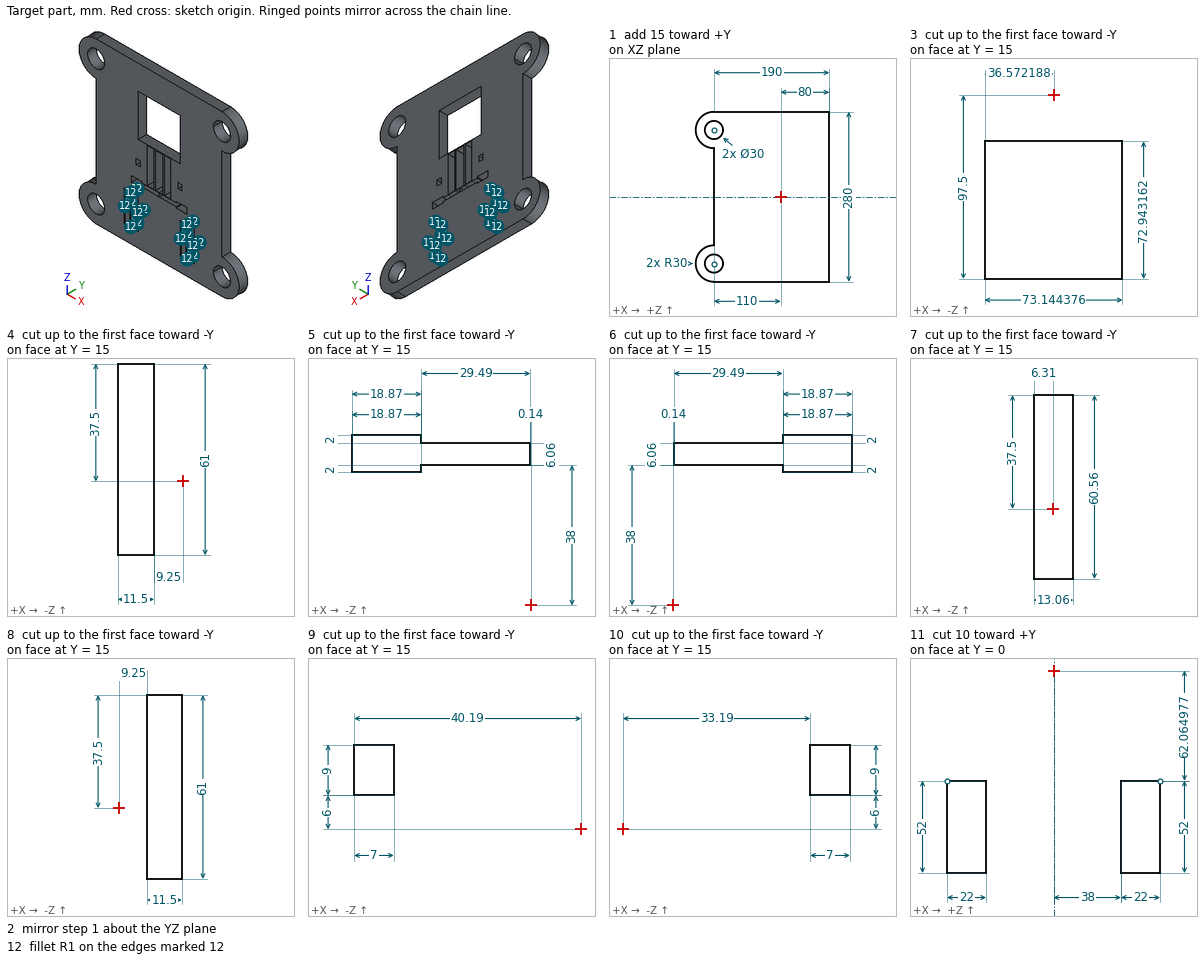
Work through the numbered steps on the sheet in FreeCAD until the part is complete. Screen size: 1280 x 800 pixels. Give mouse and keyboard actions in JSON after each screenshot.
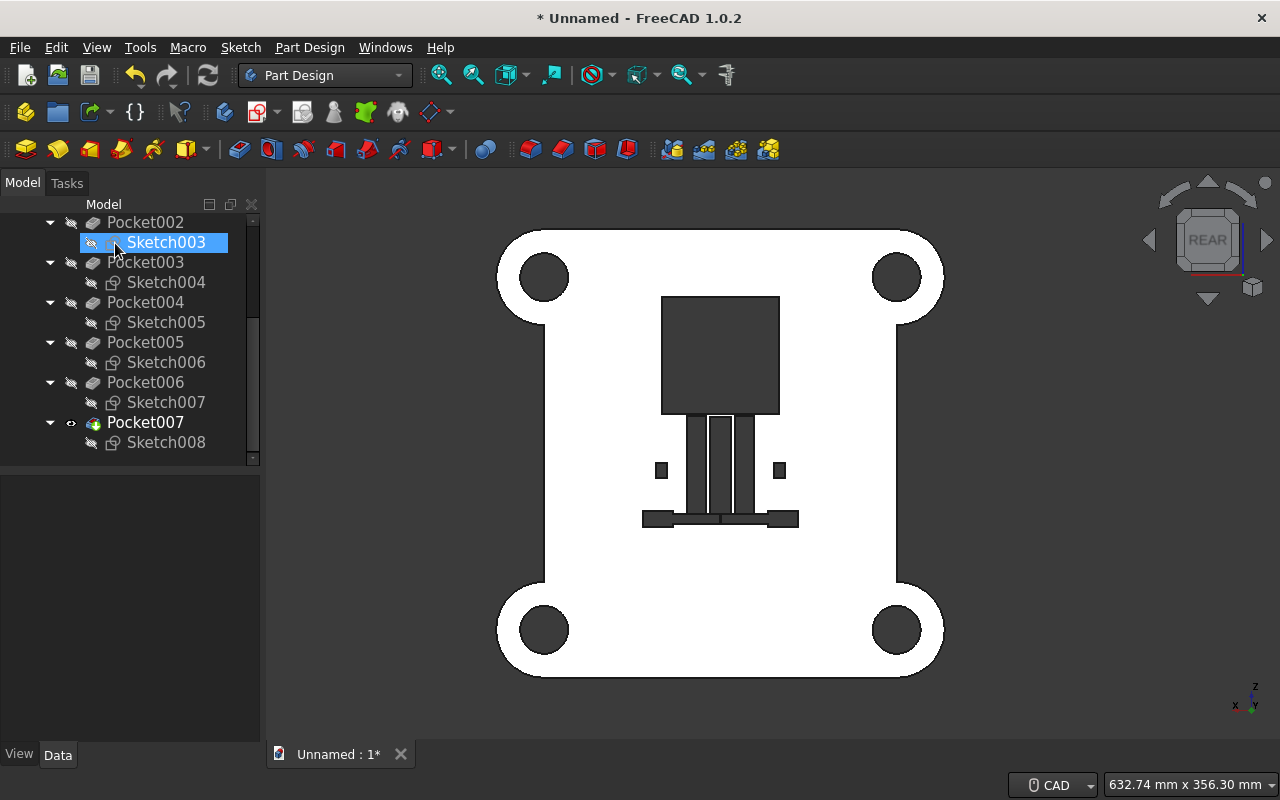
{"action": "key", "text": "0"}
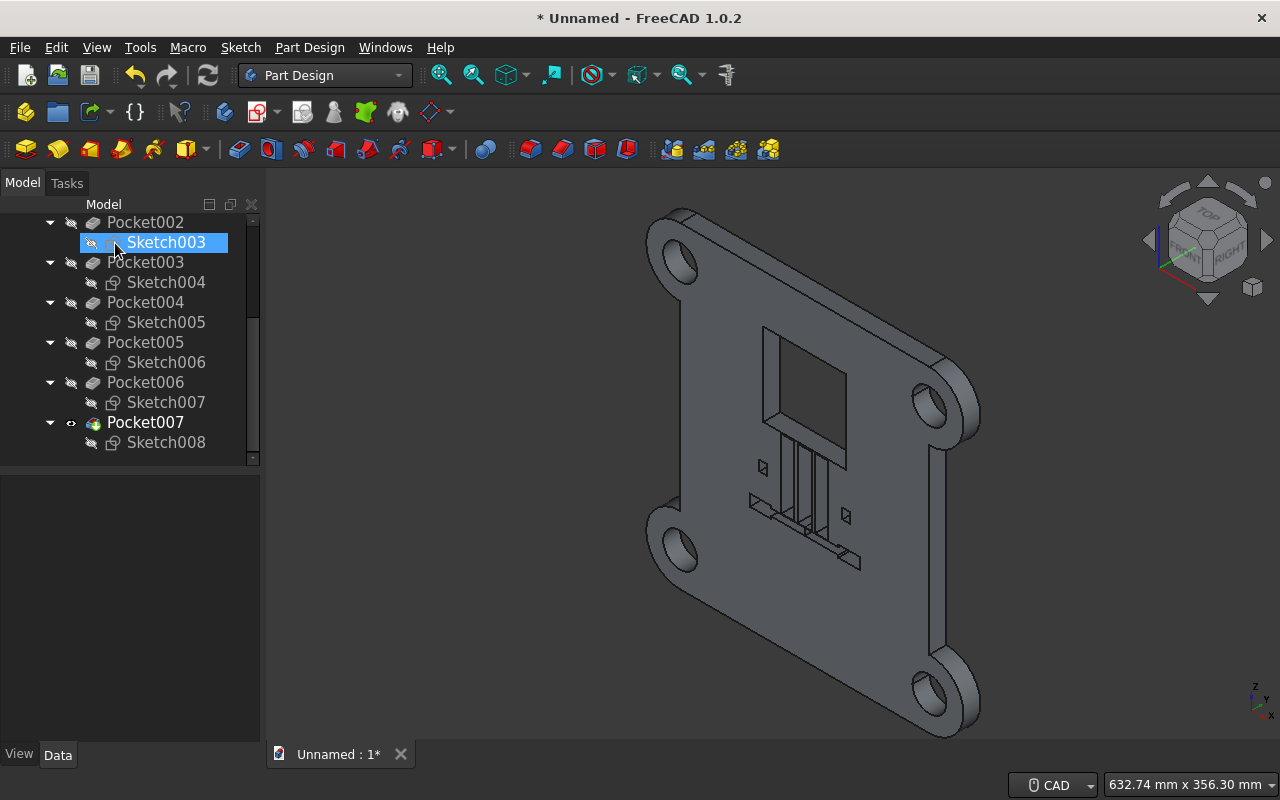
{"action": "left_click", "coordinate": [442, 76]}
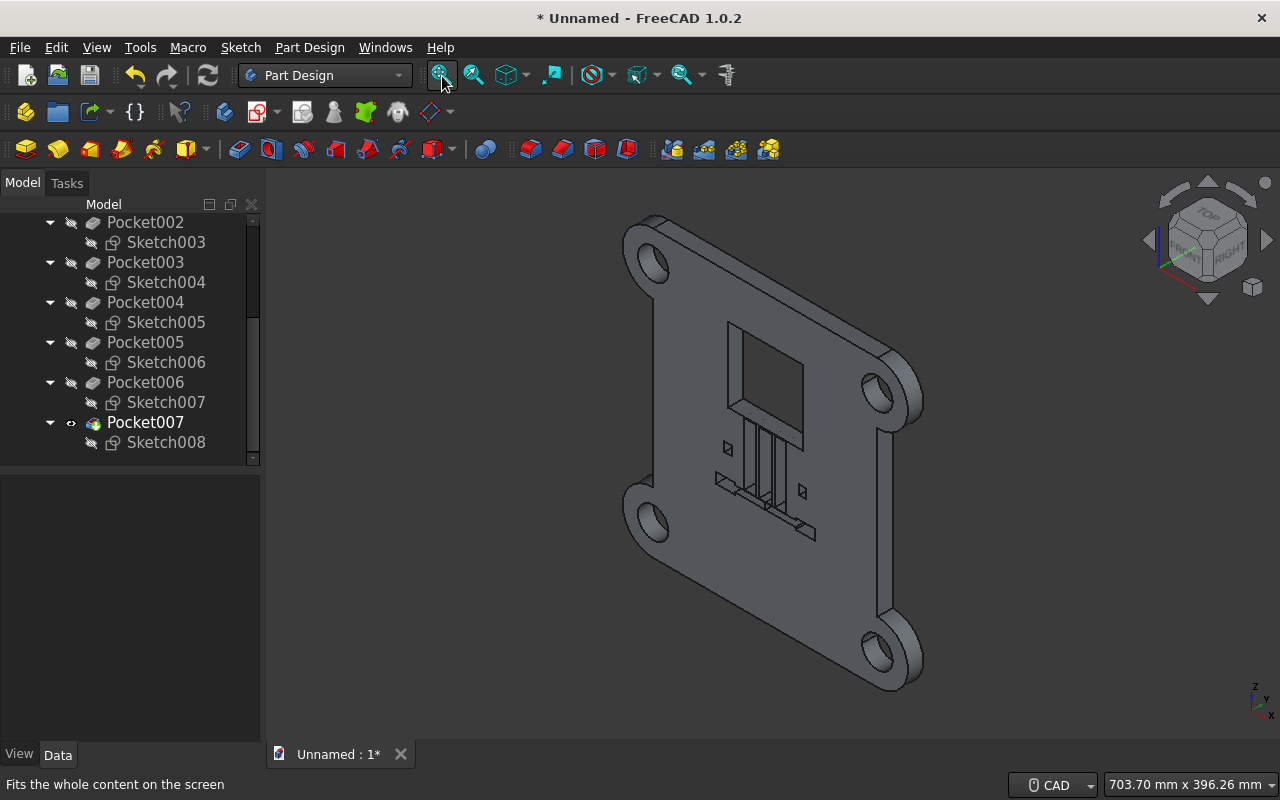
{"action": "left_click", "coordinate": [765, 551]}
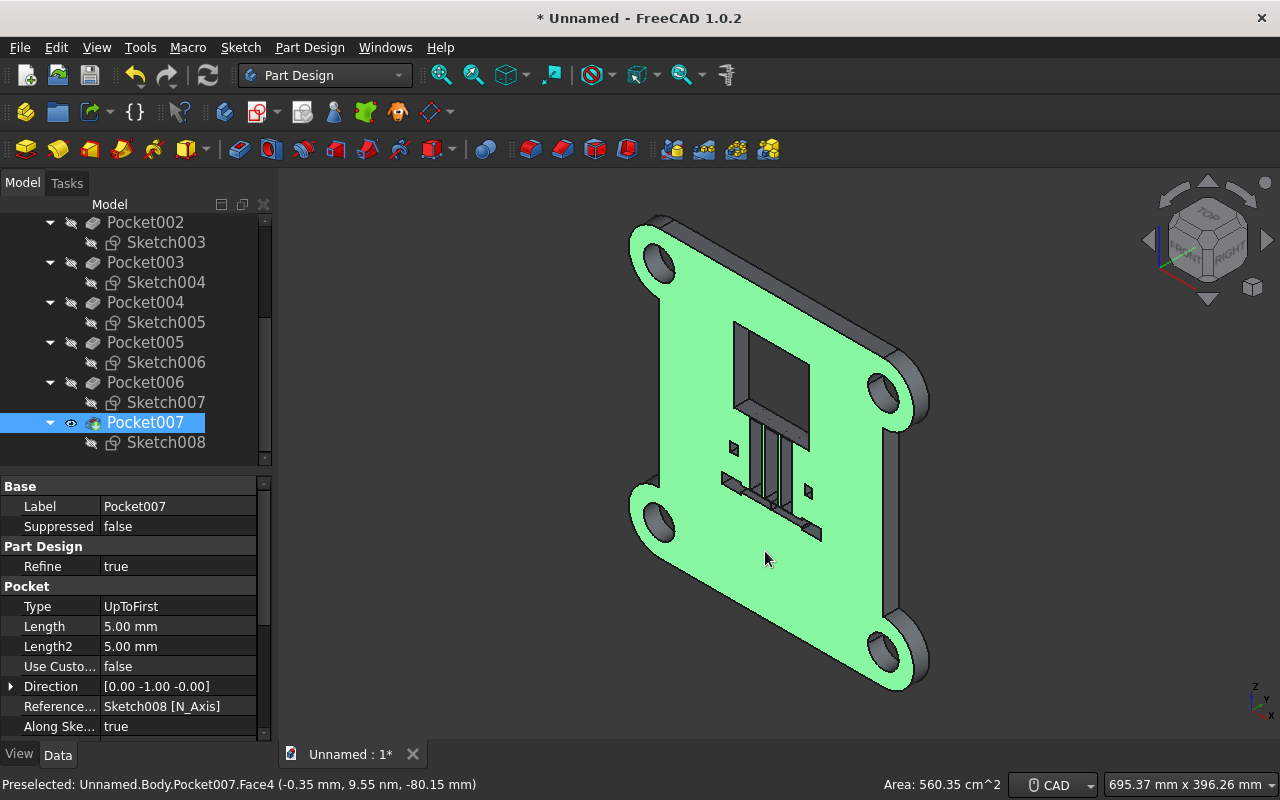
{"action": "left_click", "coordinate": [258, 112]}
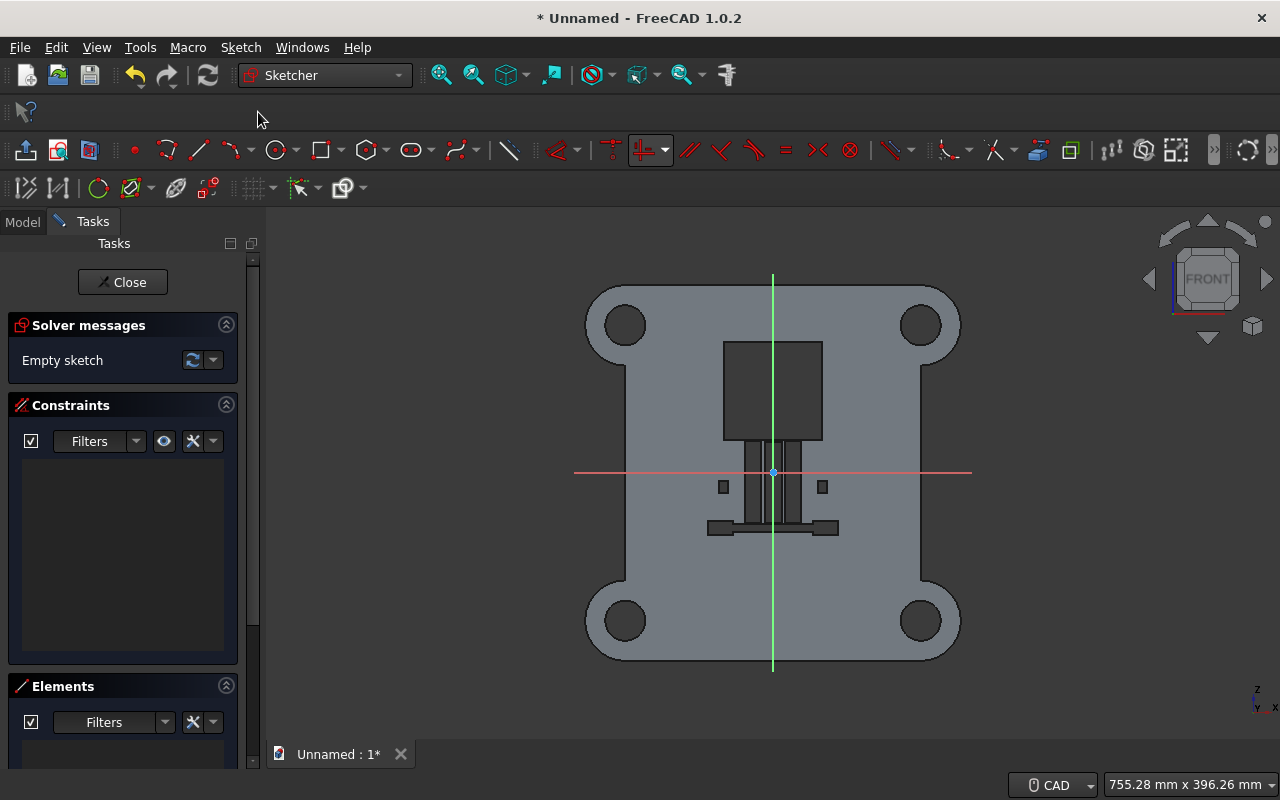
{"action": "scroll", "coordinate": [829, 612], "scroll_direction": "up", "scroll_amount": 4}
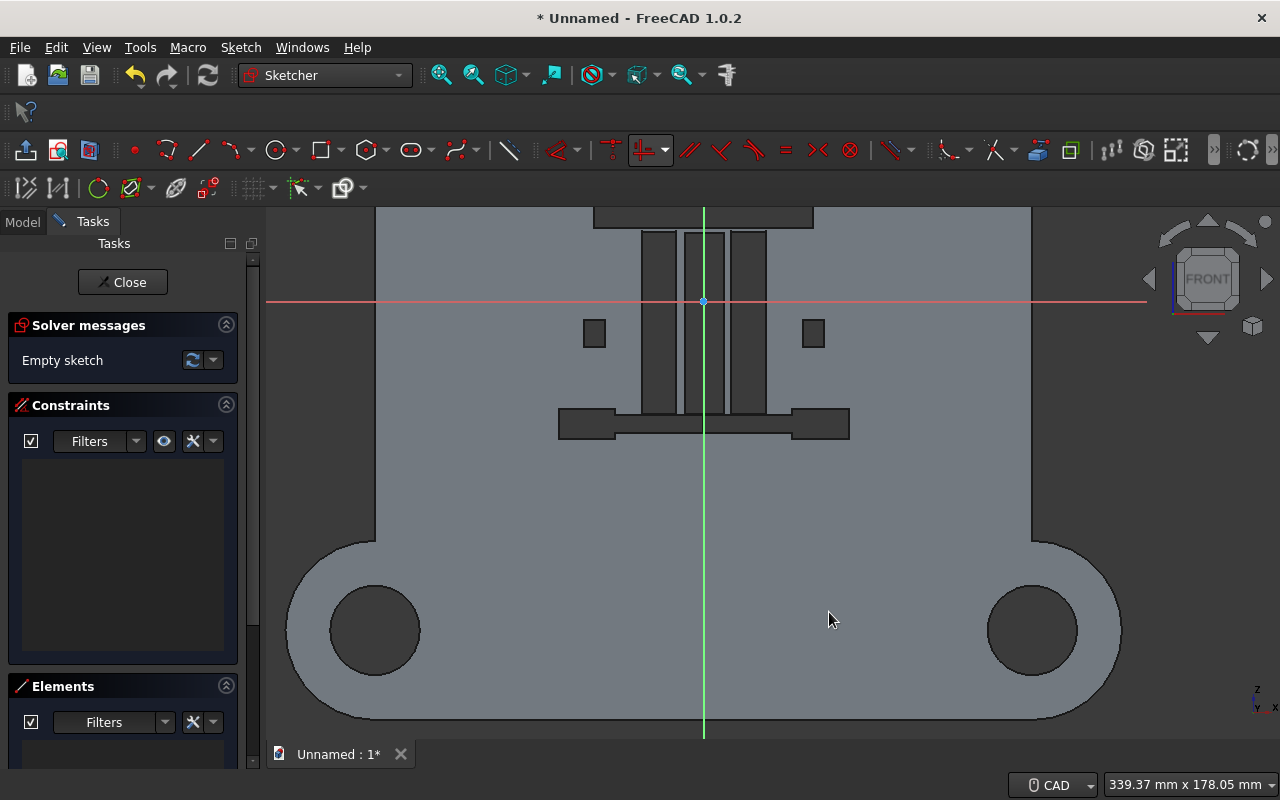
{"action": "left_click", "coordinate": [322, 150]}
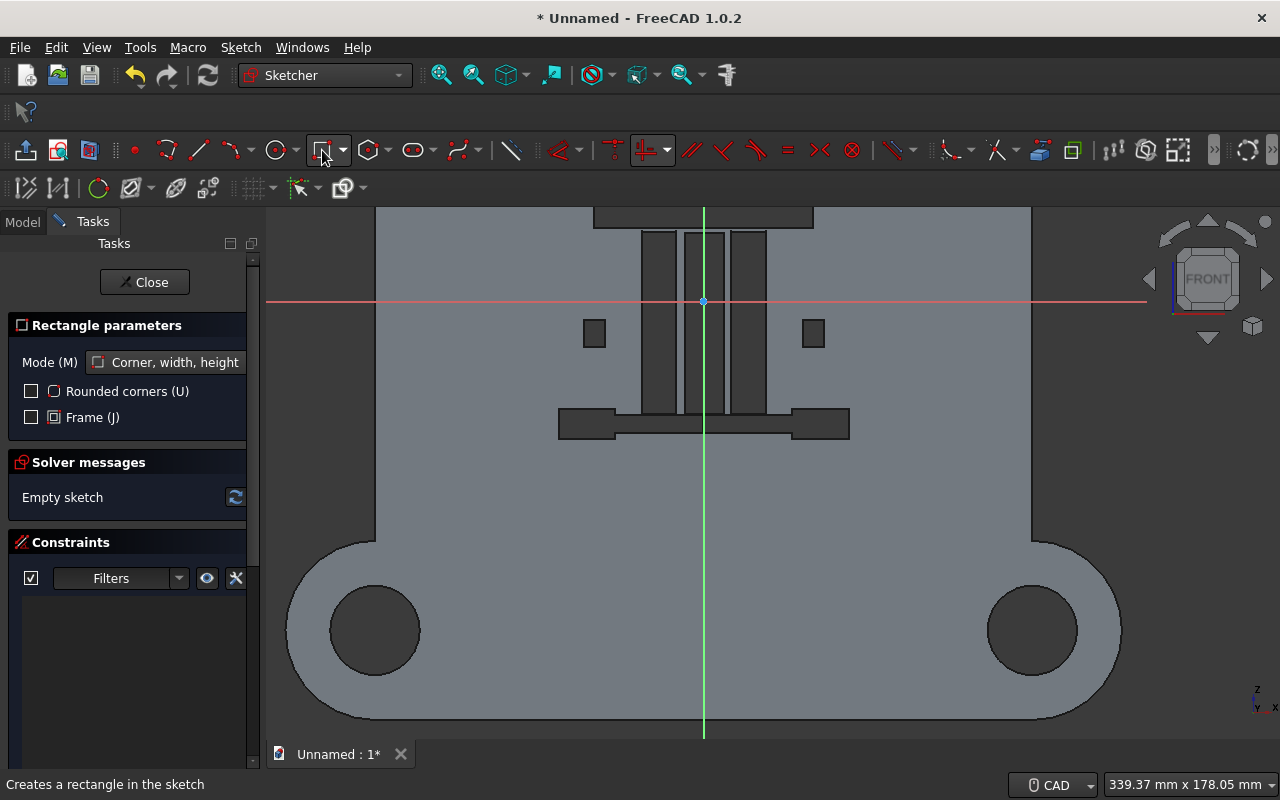
{"action": "left_click", "coordinate": [817, 487]}
{"action": "mouse_move", "coordinate": [883, 643]}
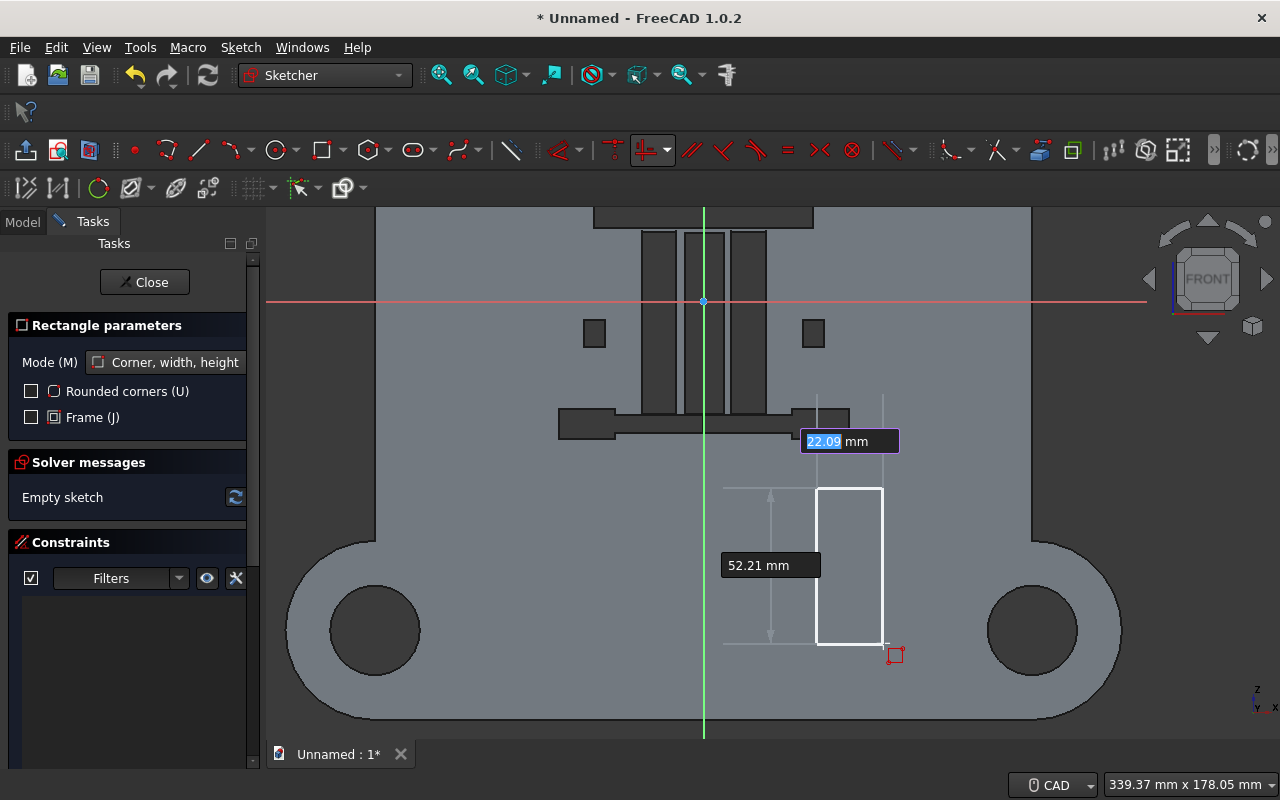
{"action": "type", "text": "22"}
{"action": "key", "text": "Tab"}
{"action": "type", "text": "52"}
{"action": "key", "text": "Return"}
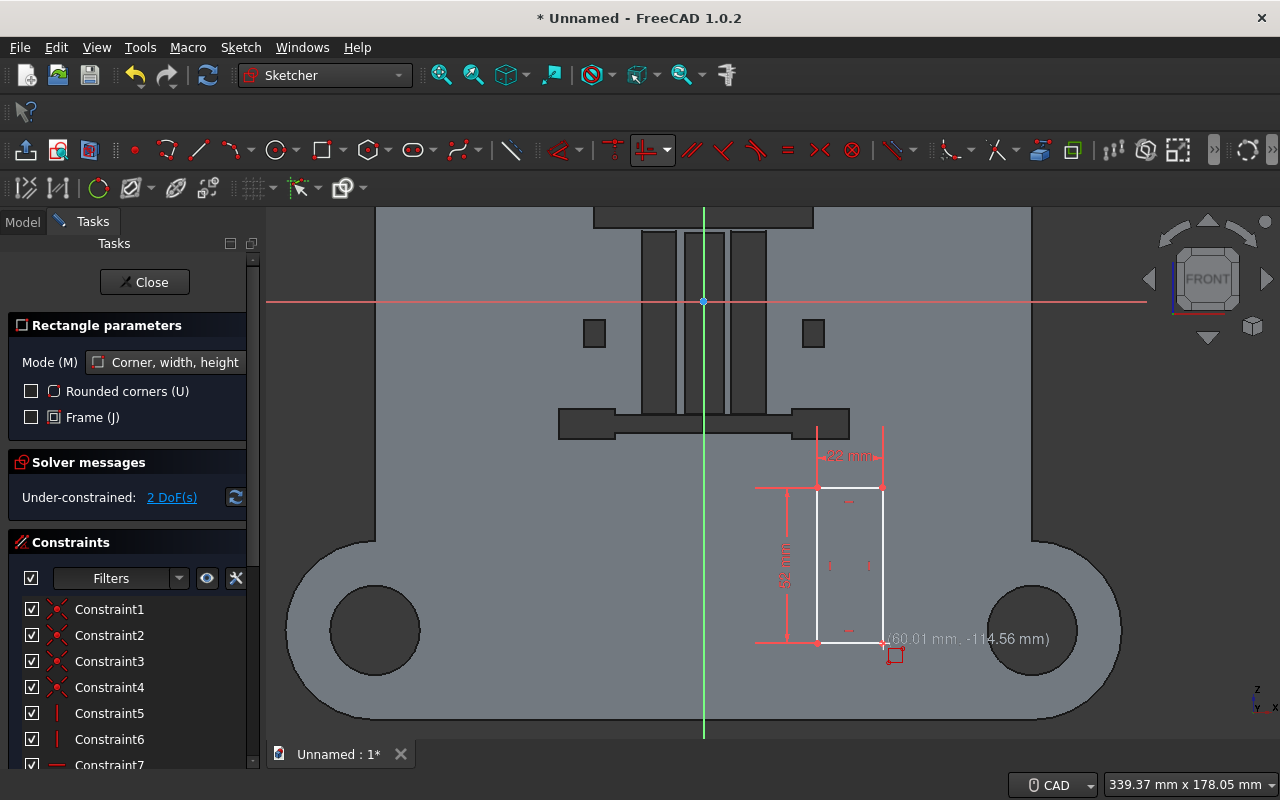
{"action": "left_click", "coordinate": [524, 487]}
{"action": "mouse_move", "coordinate": [590, 643]}